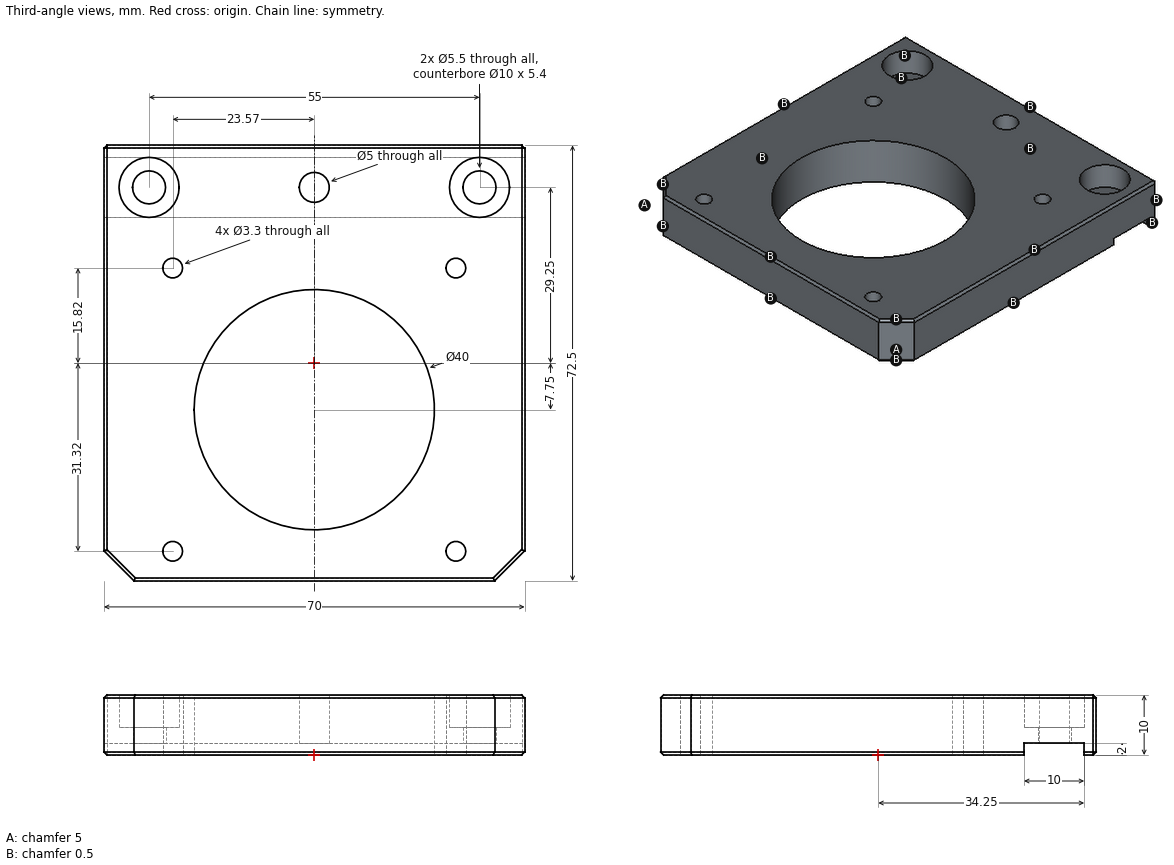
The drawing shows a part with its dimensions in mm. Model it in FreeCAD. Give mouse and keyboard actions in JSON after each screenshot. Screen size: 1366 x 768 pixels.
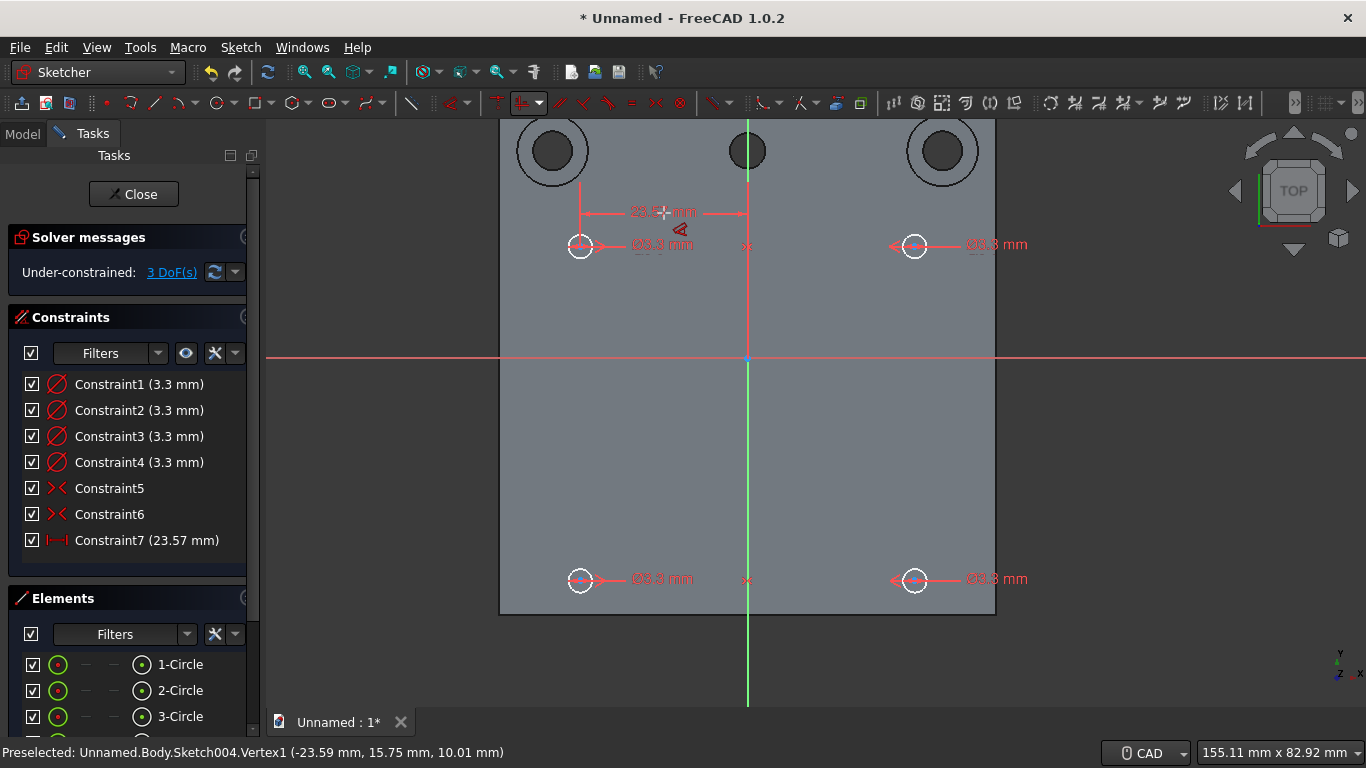
{"action": "left_click", "coordinate": [580, 247]}
{"action": "left_click", "coordinate": [546, 302]}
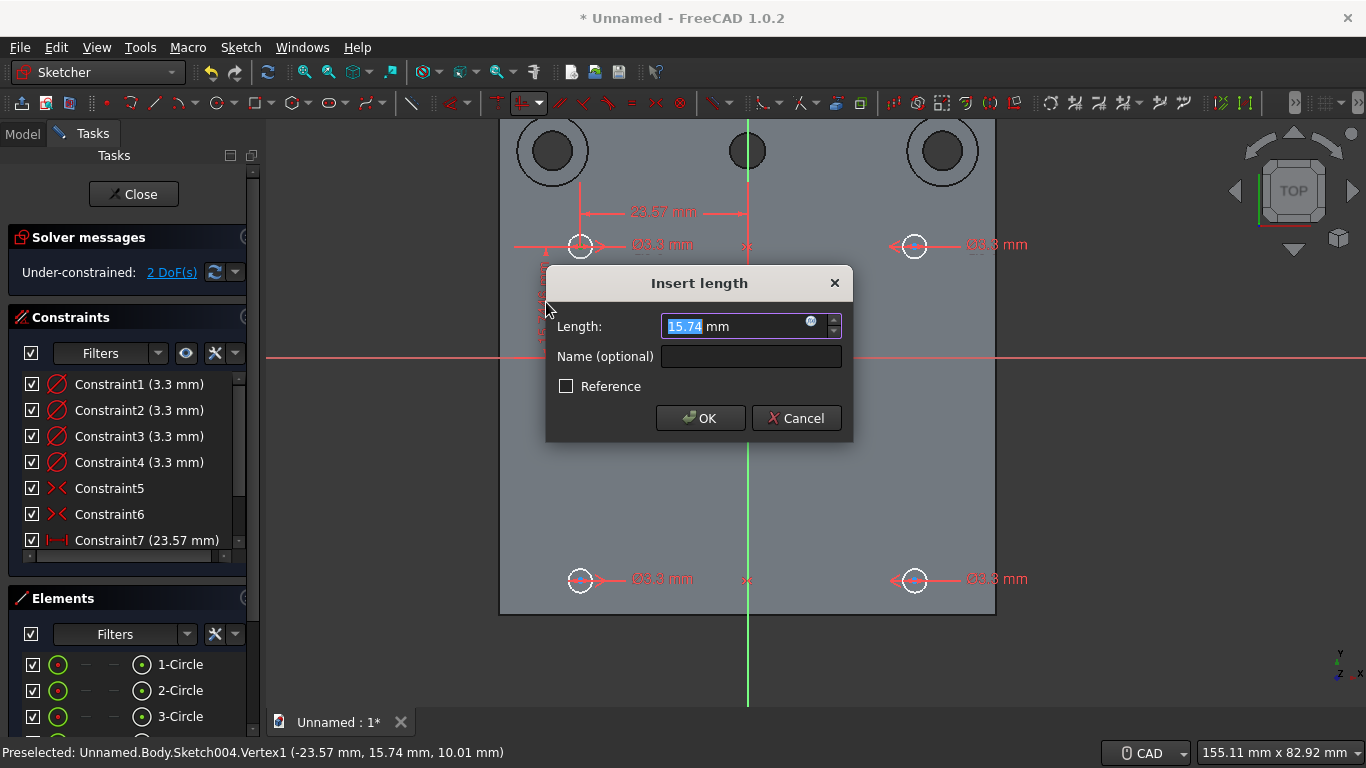
{"action": "type", "text": "15.82"}
{"action": "key", "text": "Return"}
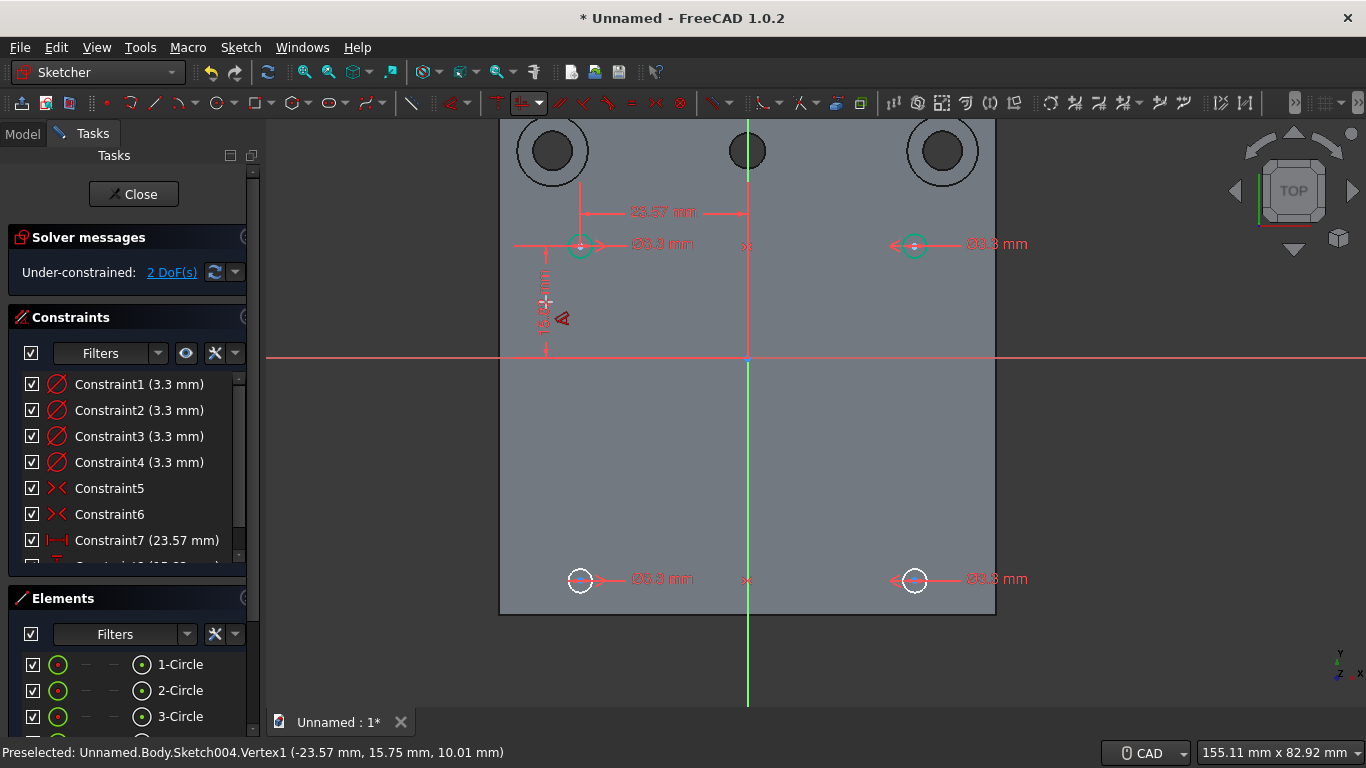
{"action": "left_click", "coordinate": [580, 581]}
{"action": "left_click", "coordinate": [664, 615]}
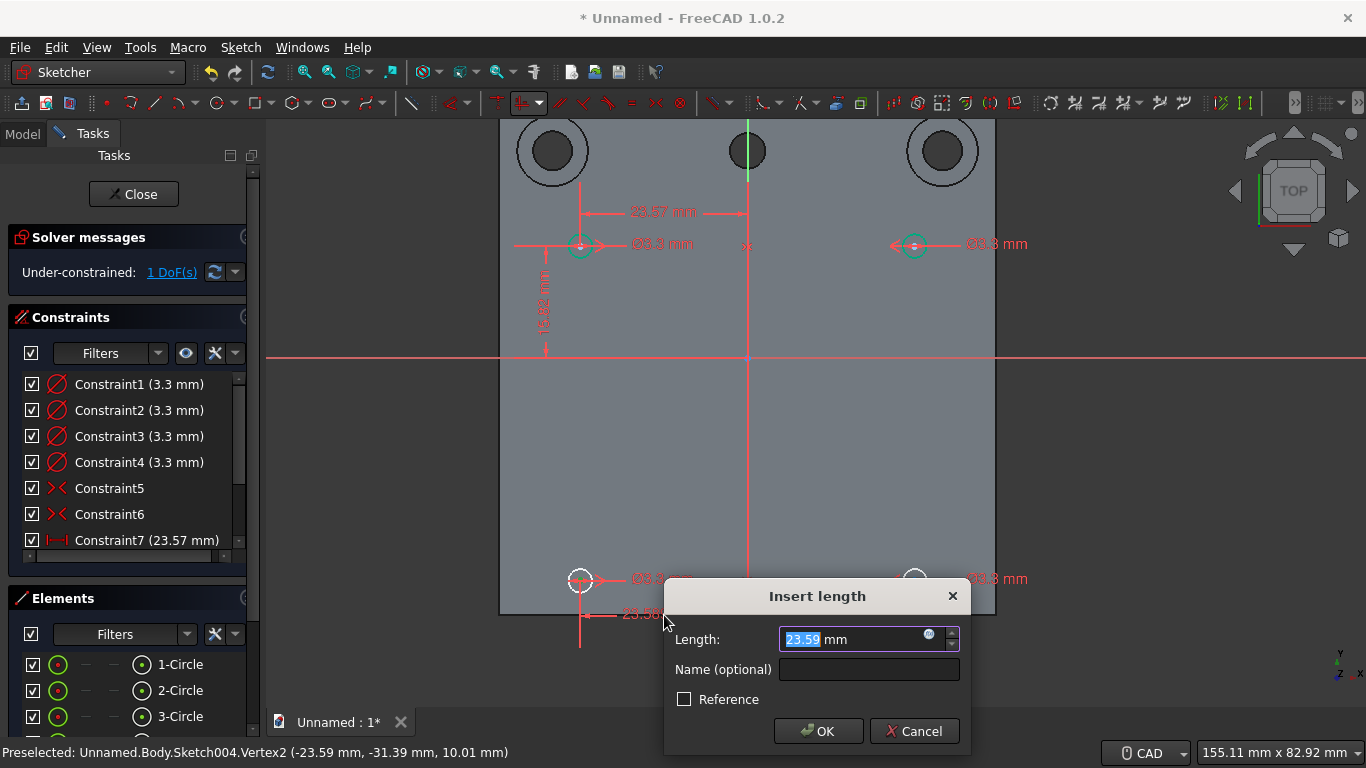
{"action": "type", "text": "23.57"}
{"action": "key", "text": "Return"}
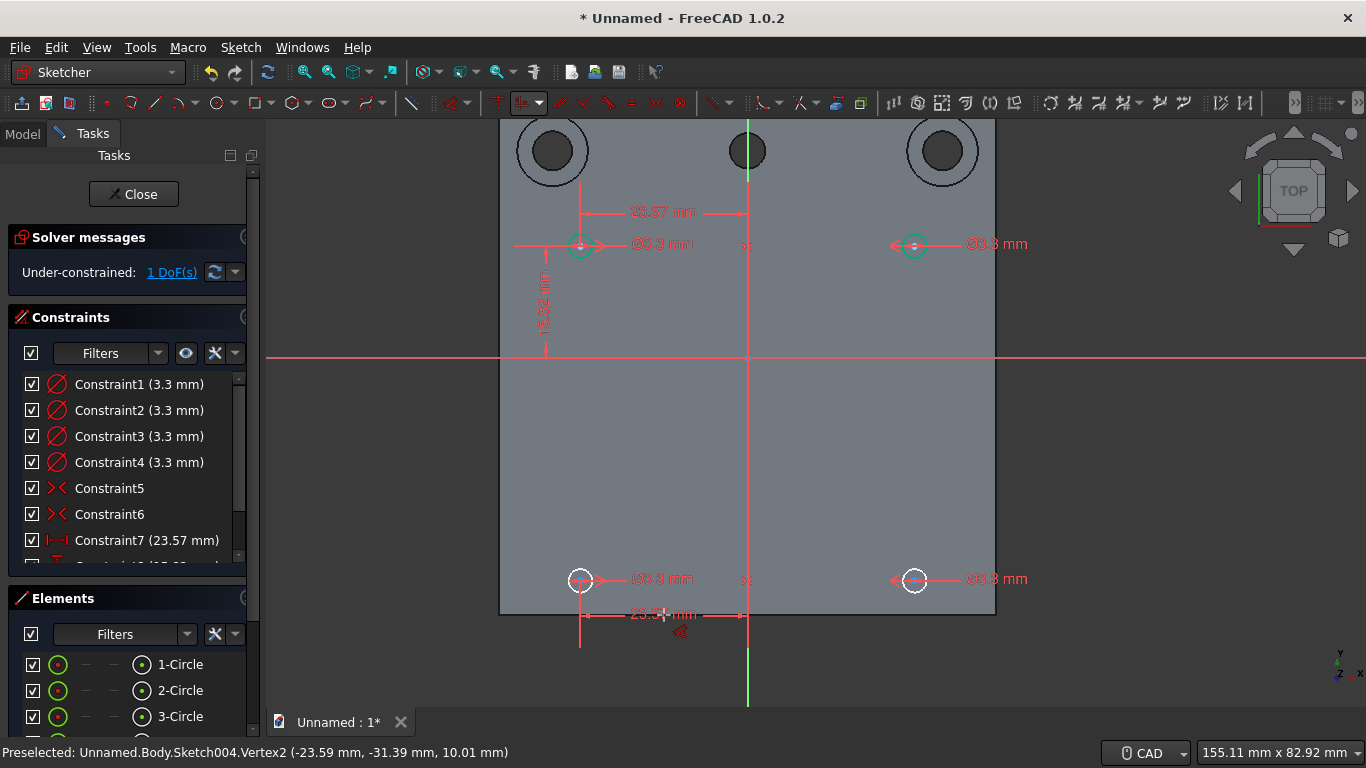
{"action": "left_click", "coordinate": [580, 581]}
{"action": "left_click", "coordinate": [546, 470]}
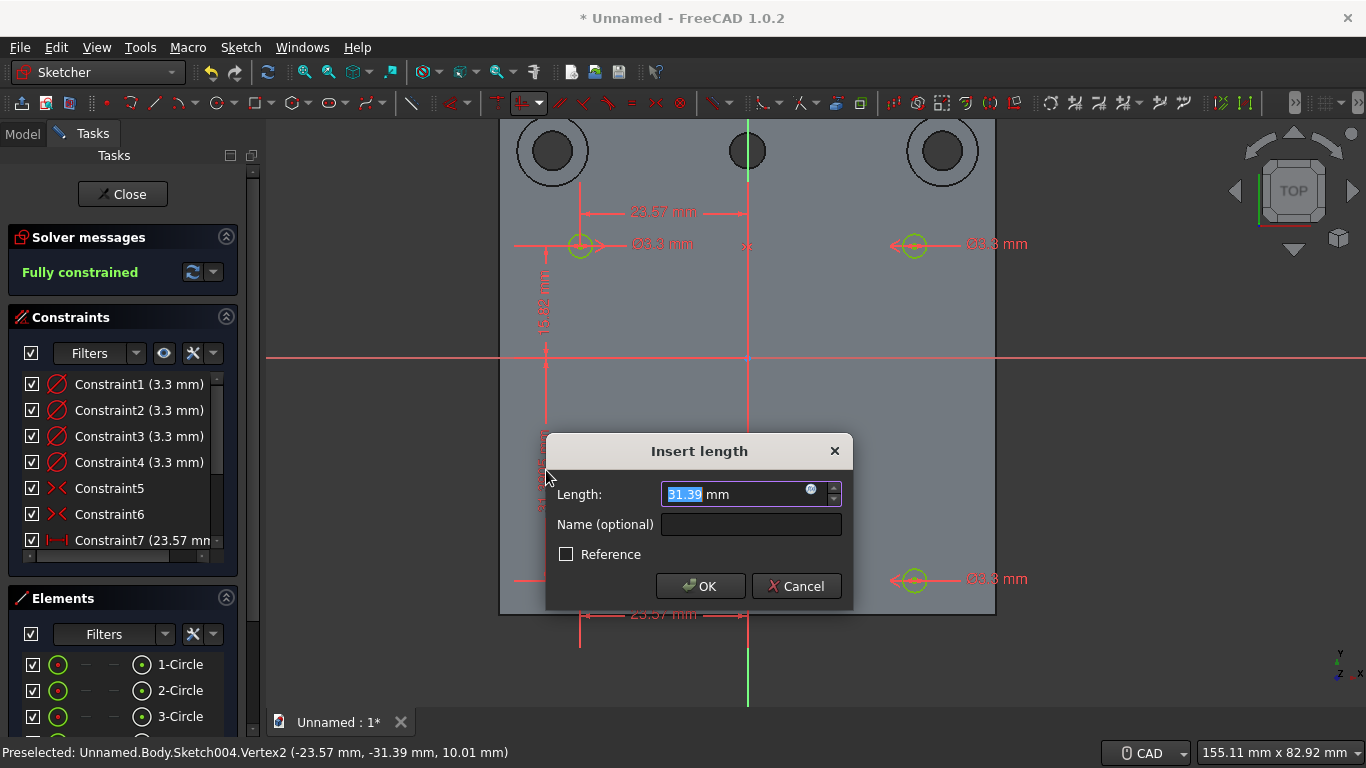
{"action": "type", "text": "31.32"}
{"action": "key", "text": "Return"}
{"action": "key", "text": "Escape"}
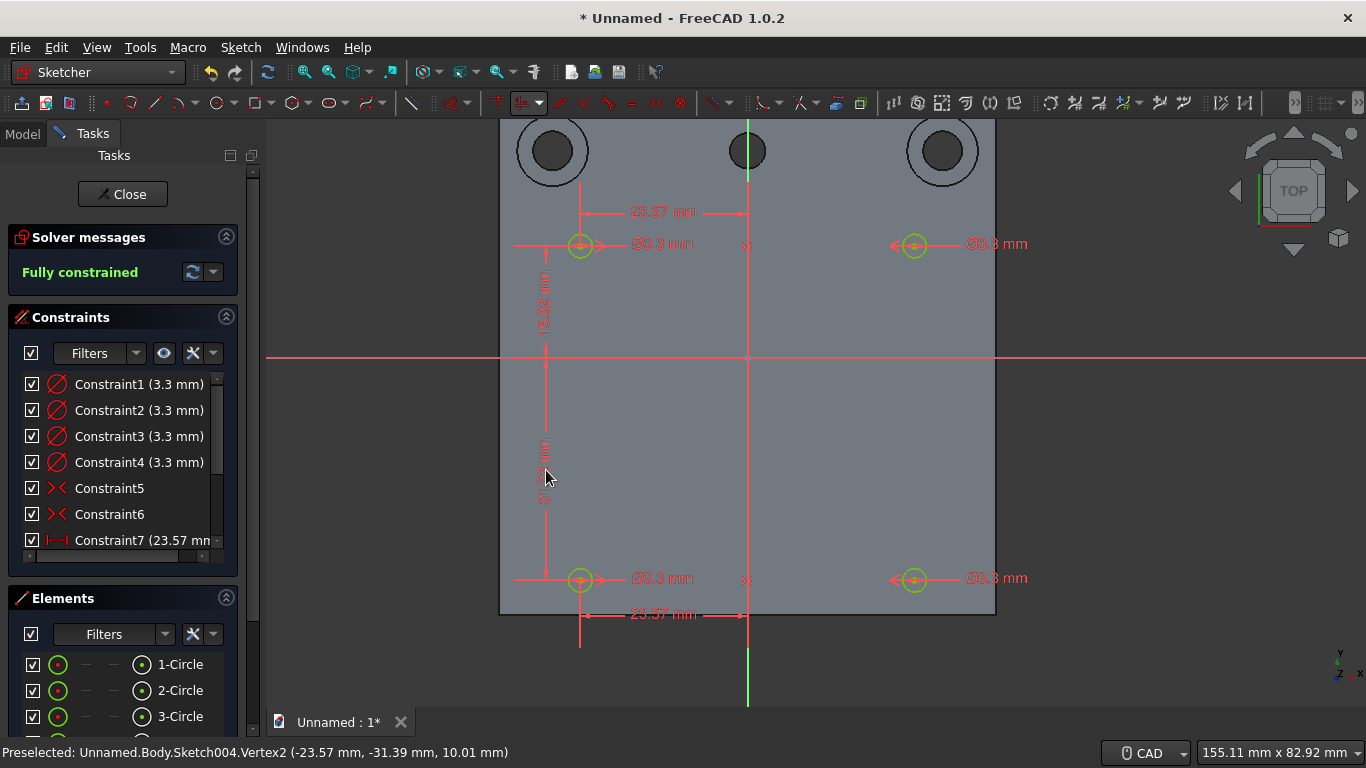
{"action": "left_click", "coordinate": [123, 194]}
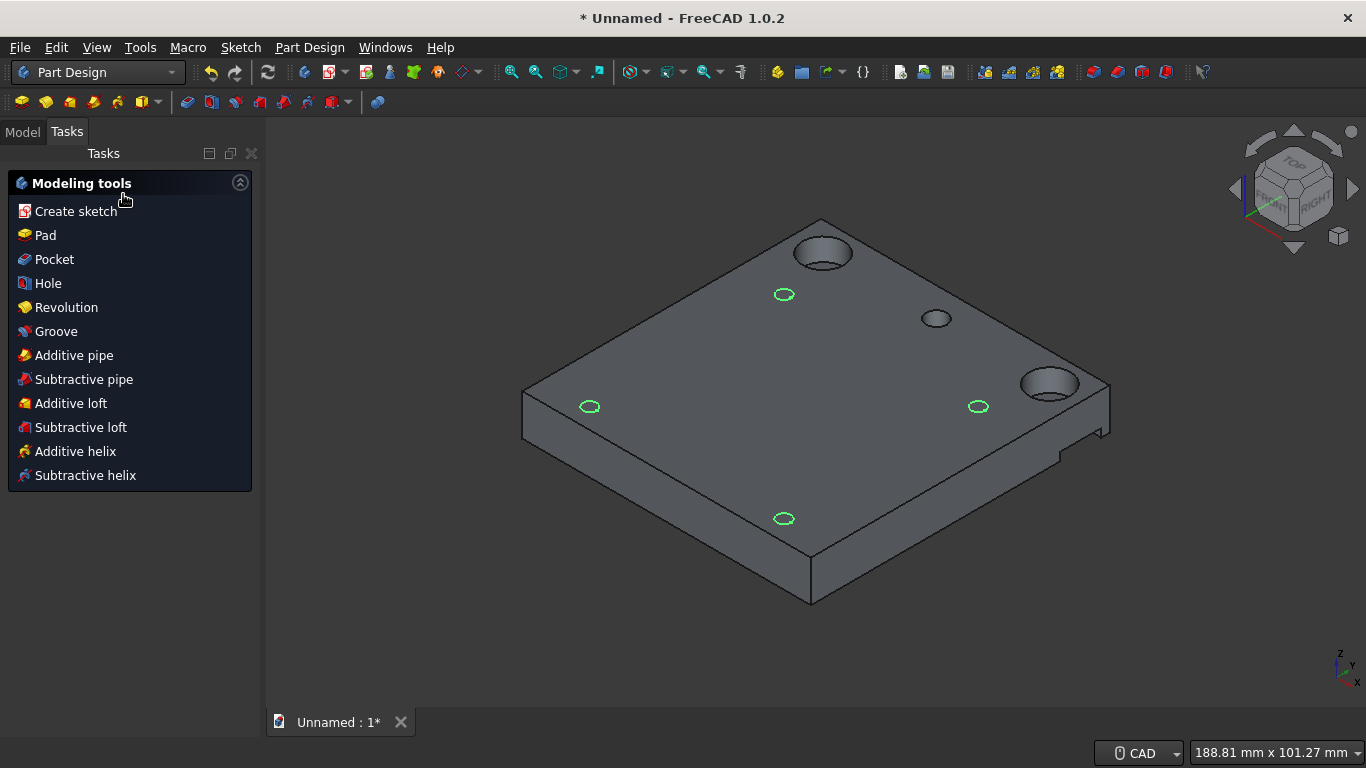
{"action": "left_click", "coordinate": [212, 102]}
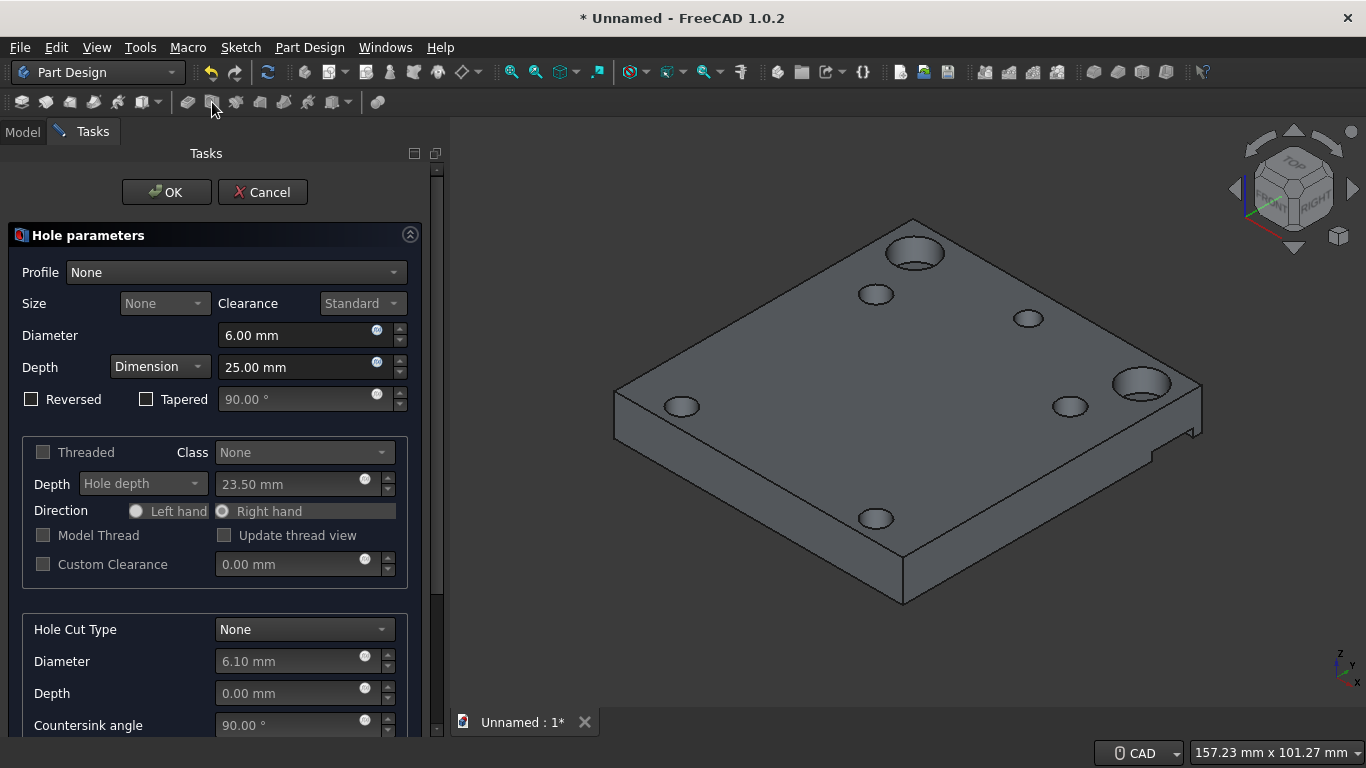
{"action": "triple_click", "coordinate": [305, 335]}